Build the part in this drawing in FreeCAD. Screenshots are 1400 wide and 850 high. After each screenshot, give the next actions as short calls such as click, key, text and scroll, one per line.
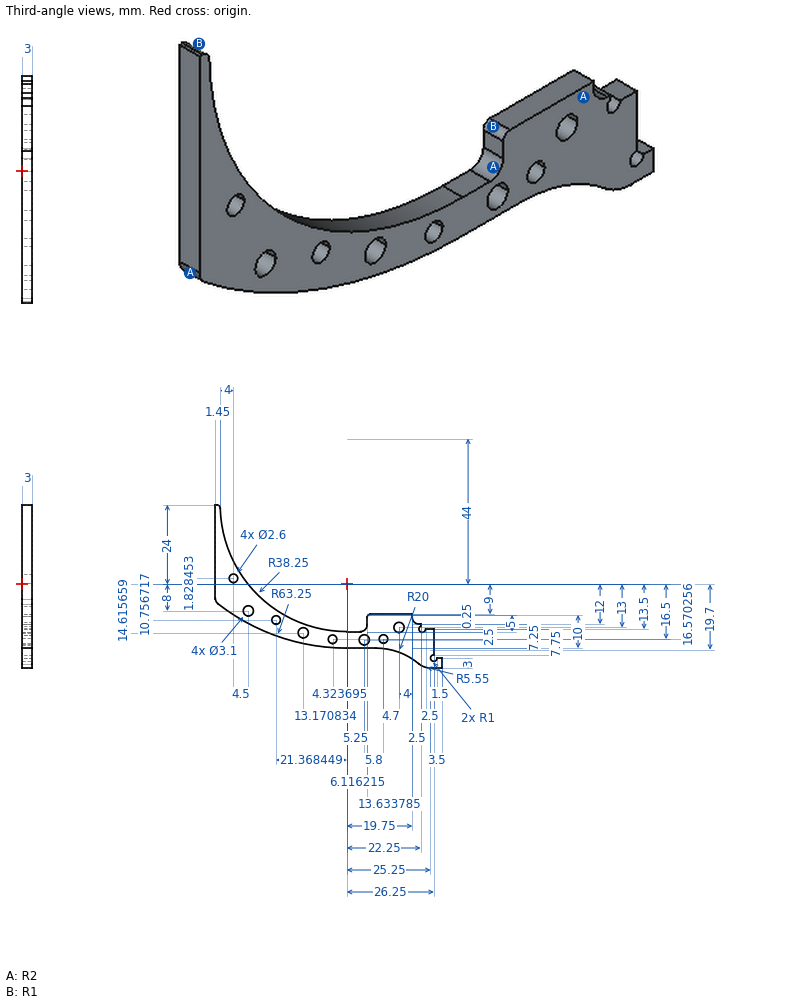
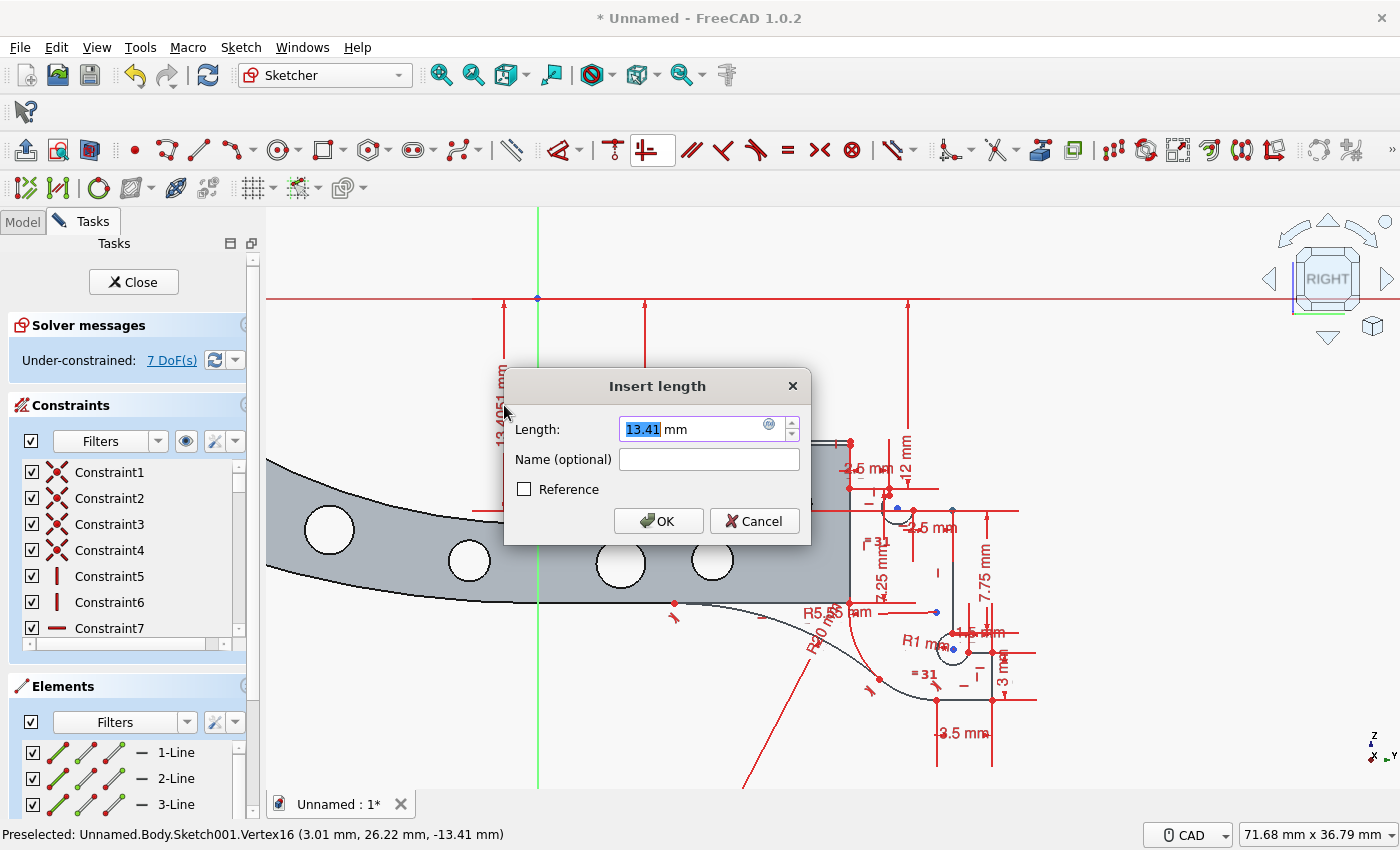
text(13.5)
key(Return)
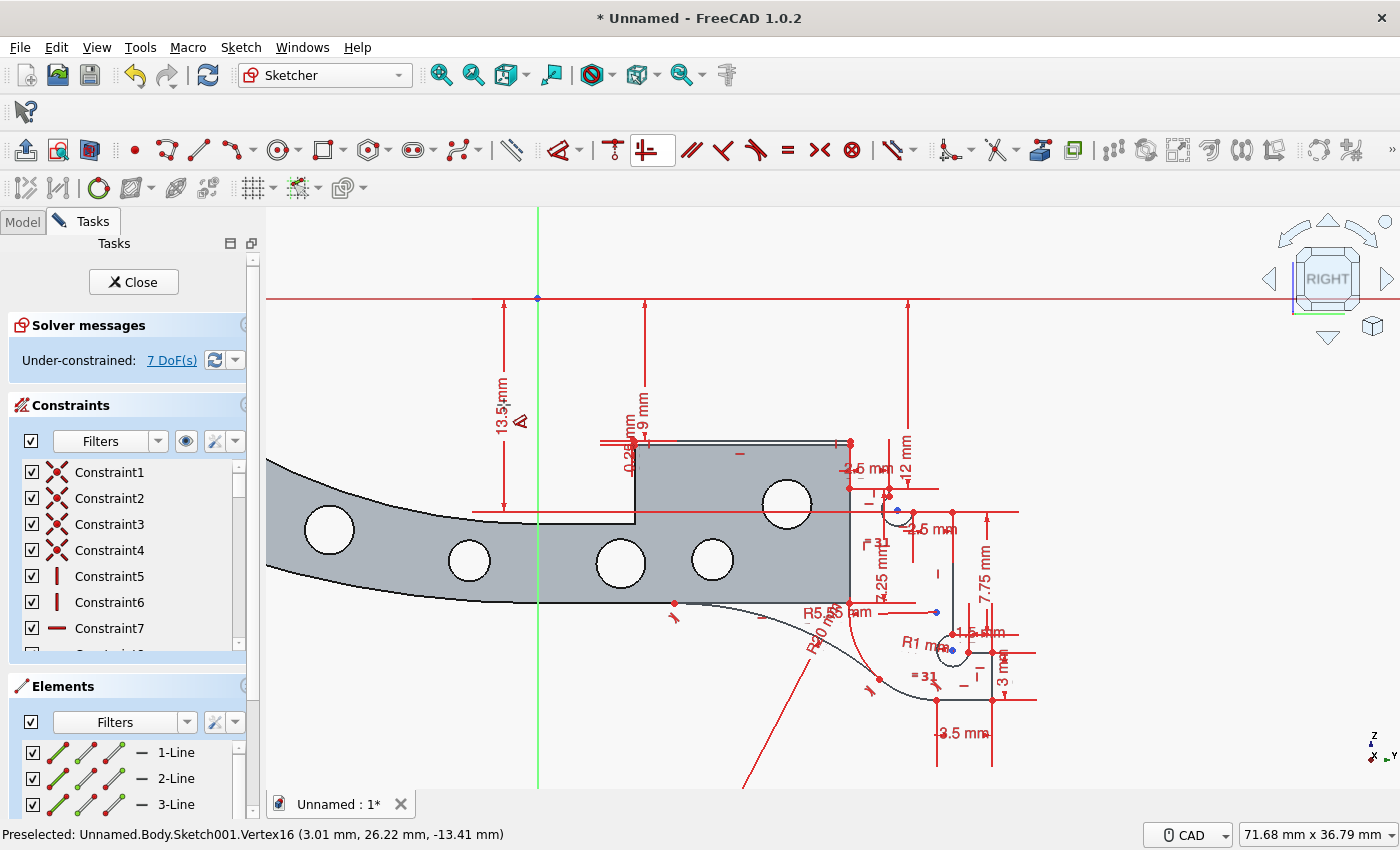
click(897, 510)
click(504, 356)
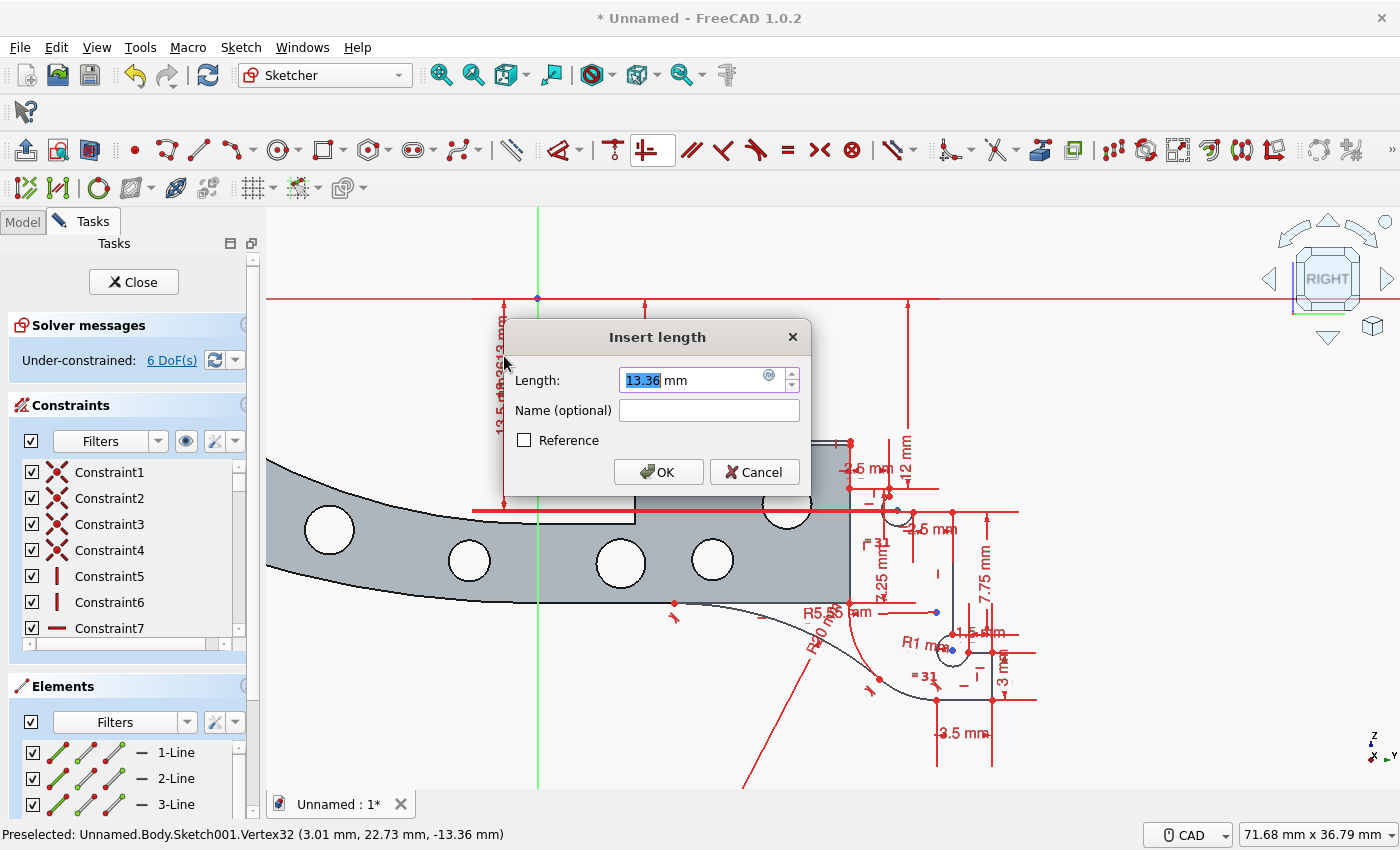
text(13.5)
key(Return)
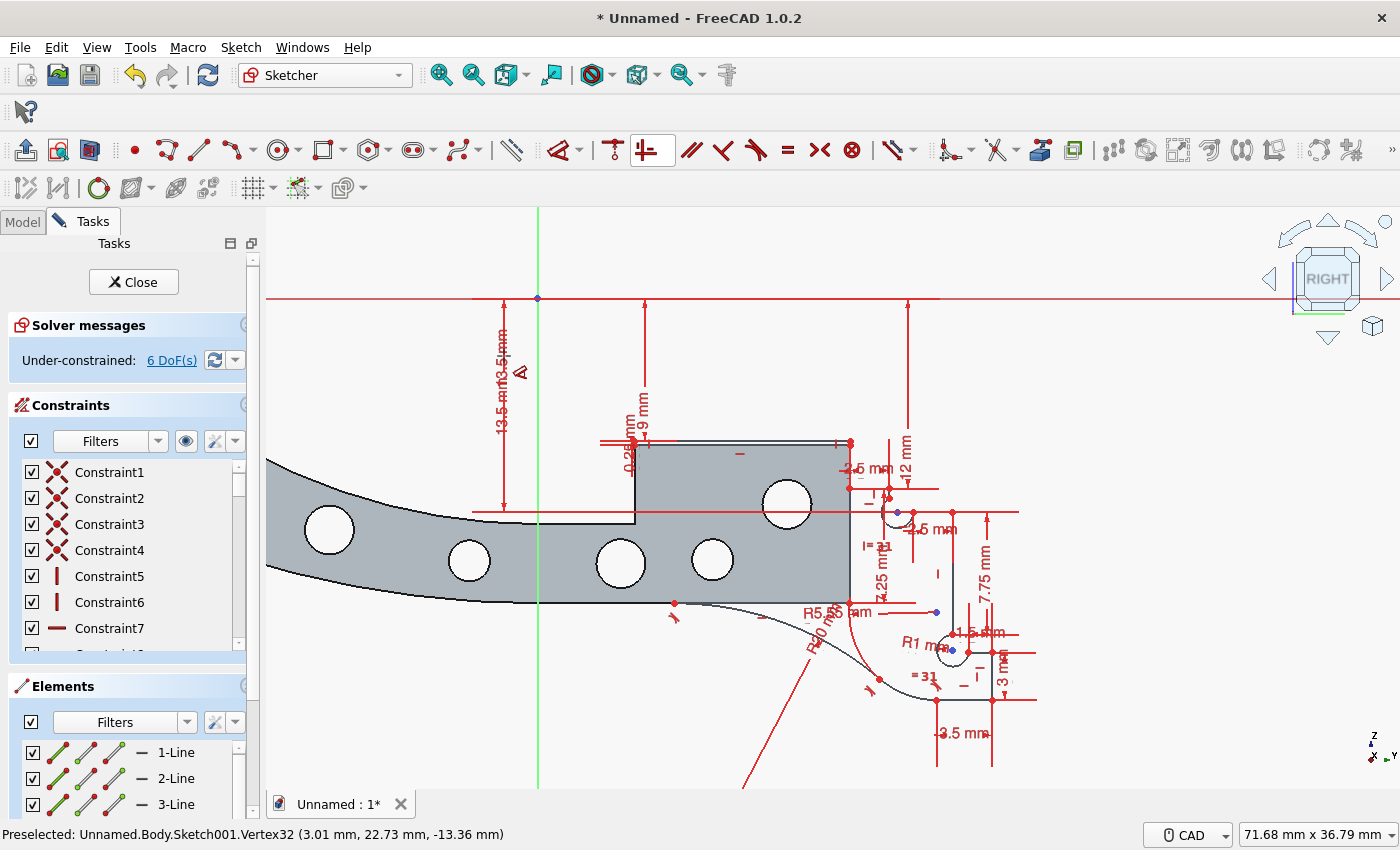
click(937, 612)
click(504, 455)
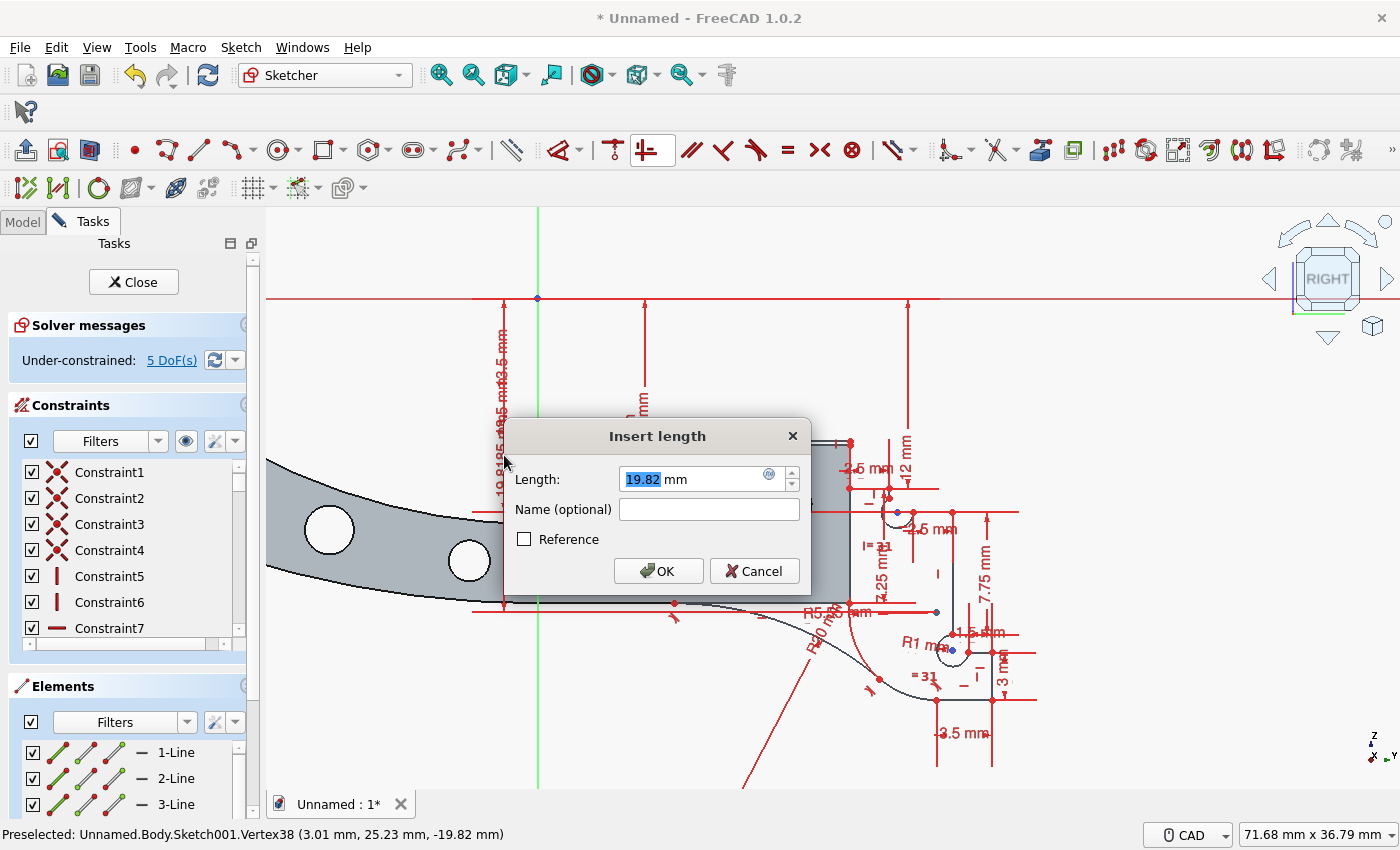
text(19.7)
key(Return)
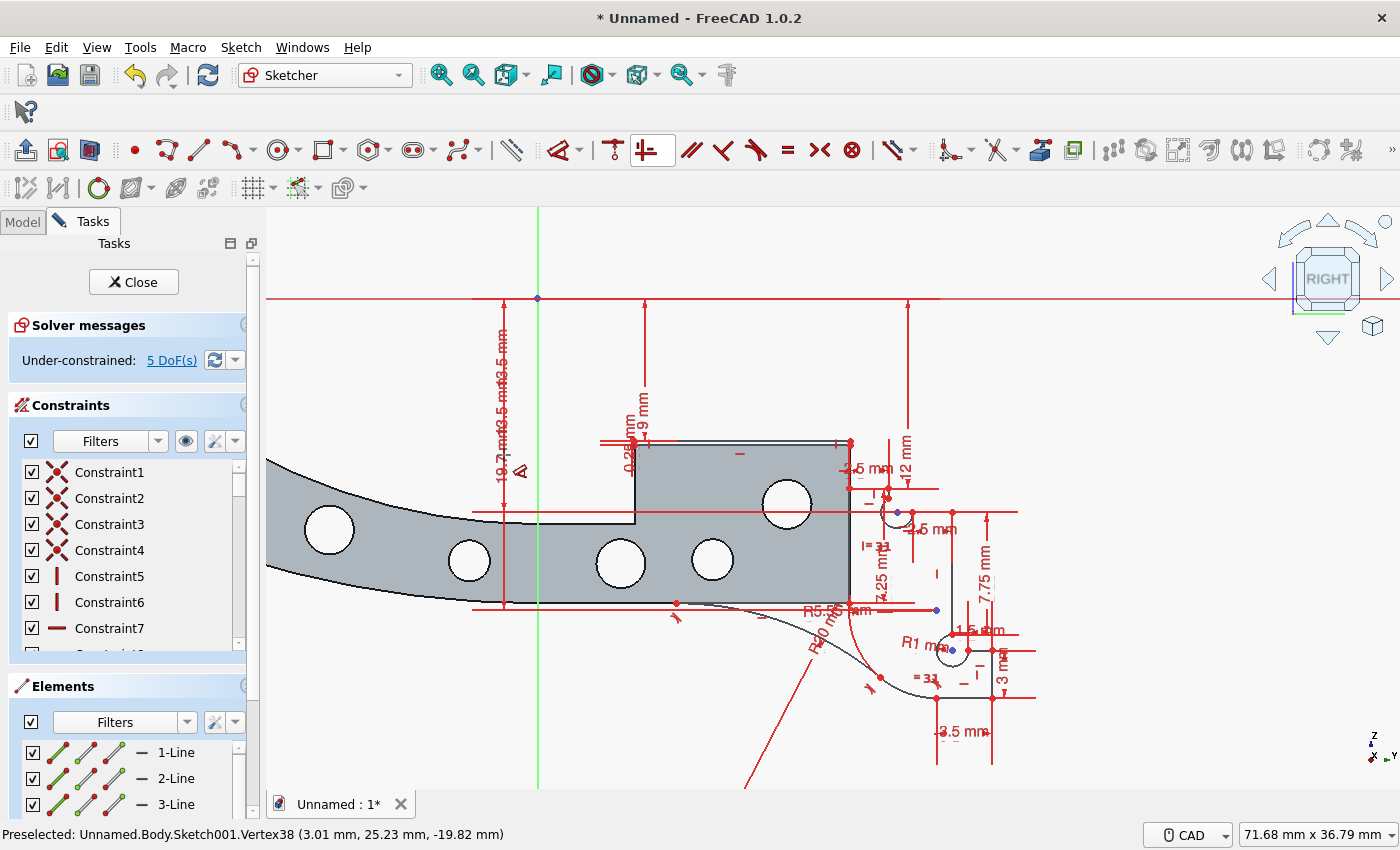
scroll(851, 445, up, 6)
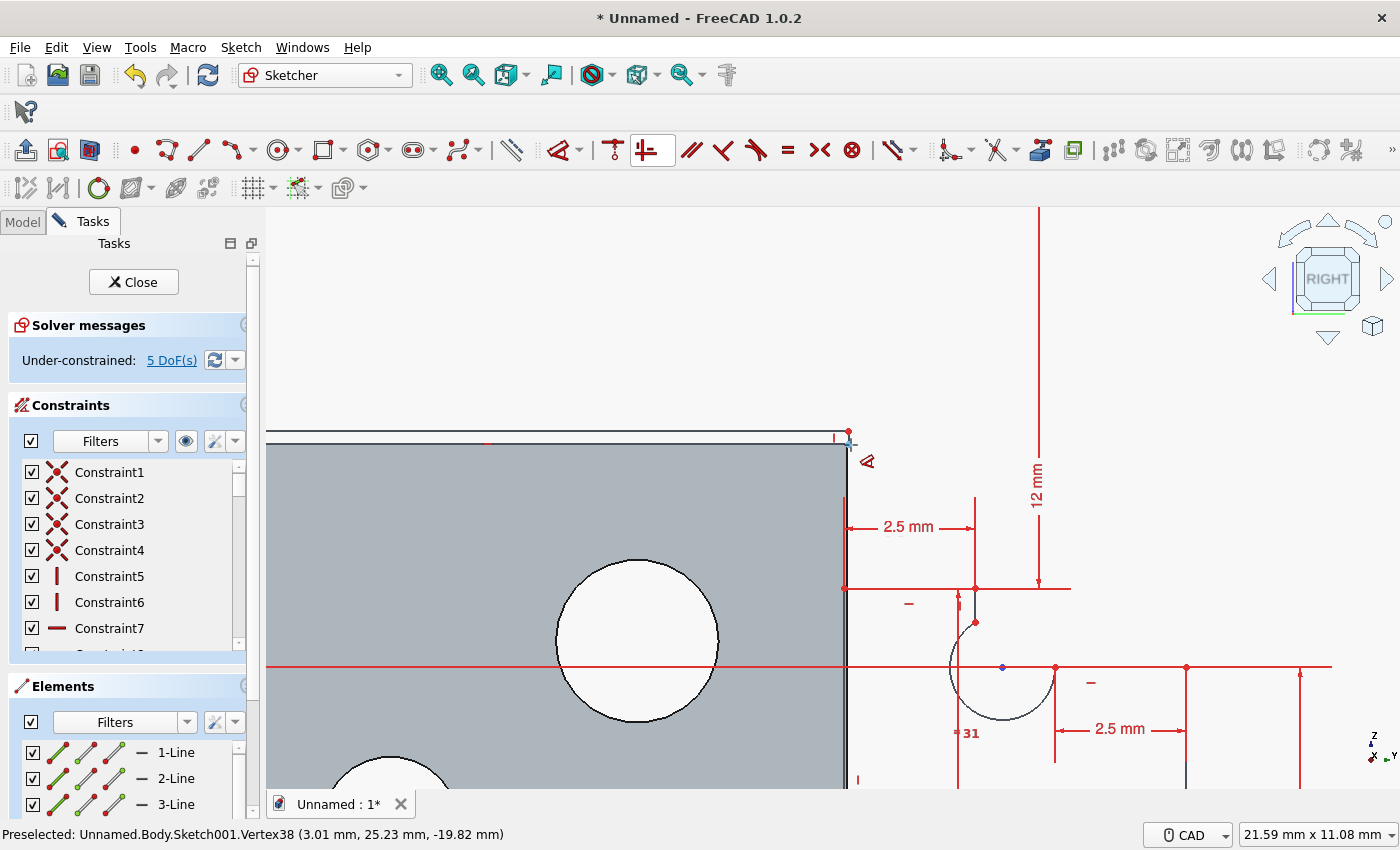
click(849, 444)
click(571, 478)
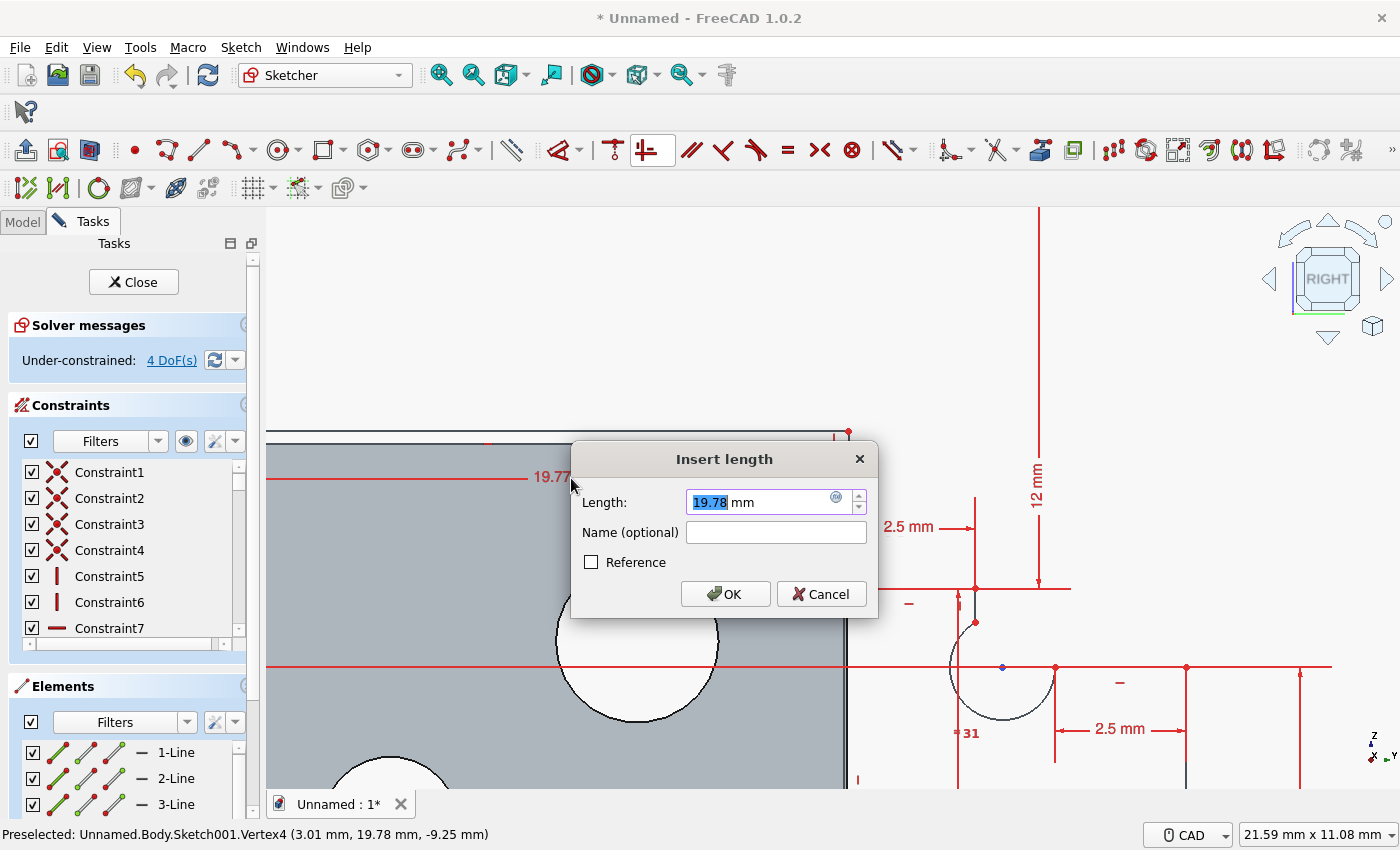
text(19.75)
key(Return)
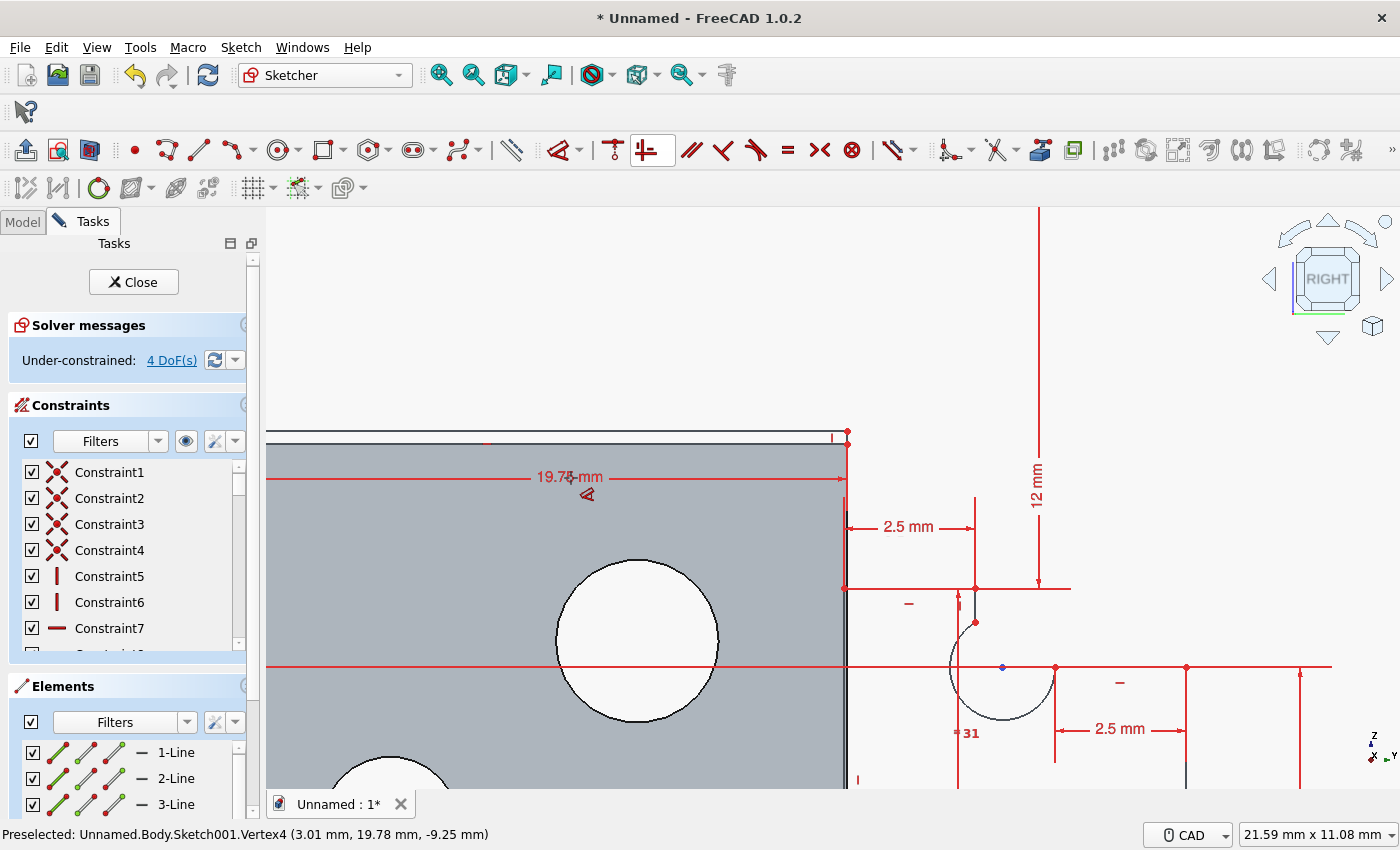
scroll(850, 445, down, 6)